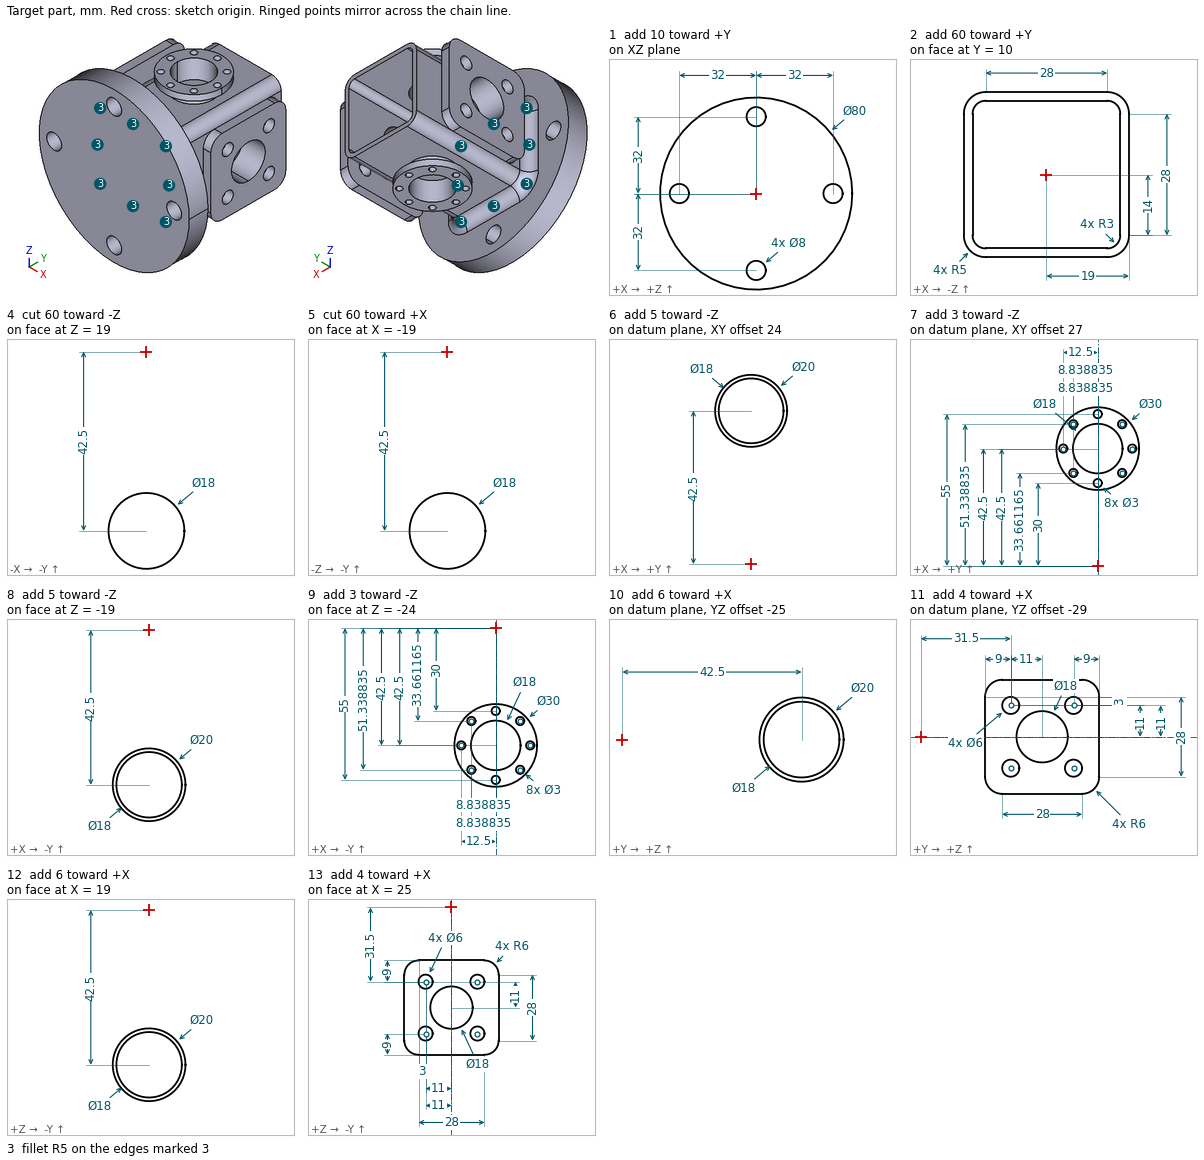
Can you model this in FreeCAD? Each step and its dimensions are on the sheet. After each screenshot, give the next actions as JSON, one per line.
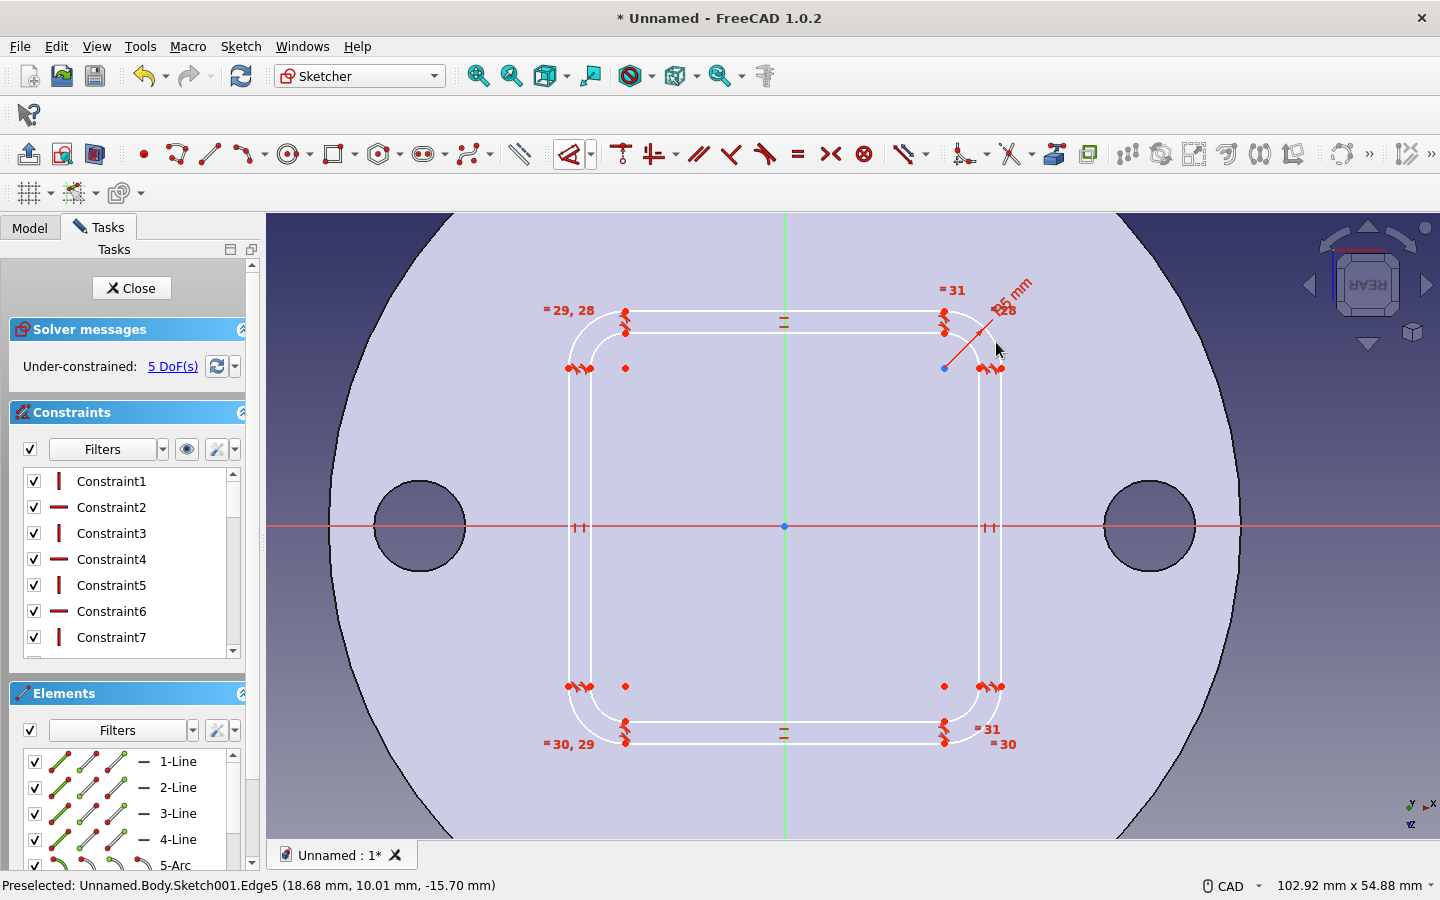
{"action": "left_click", "coordinate": [960, 718]}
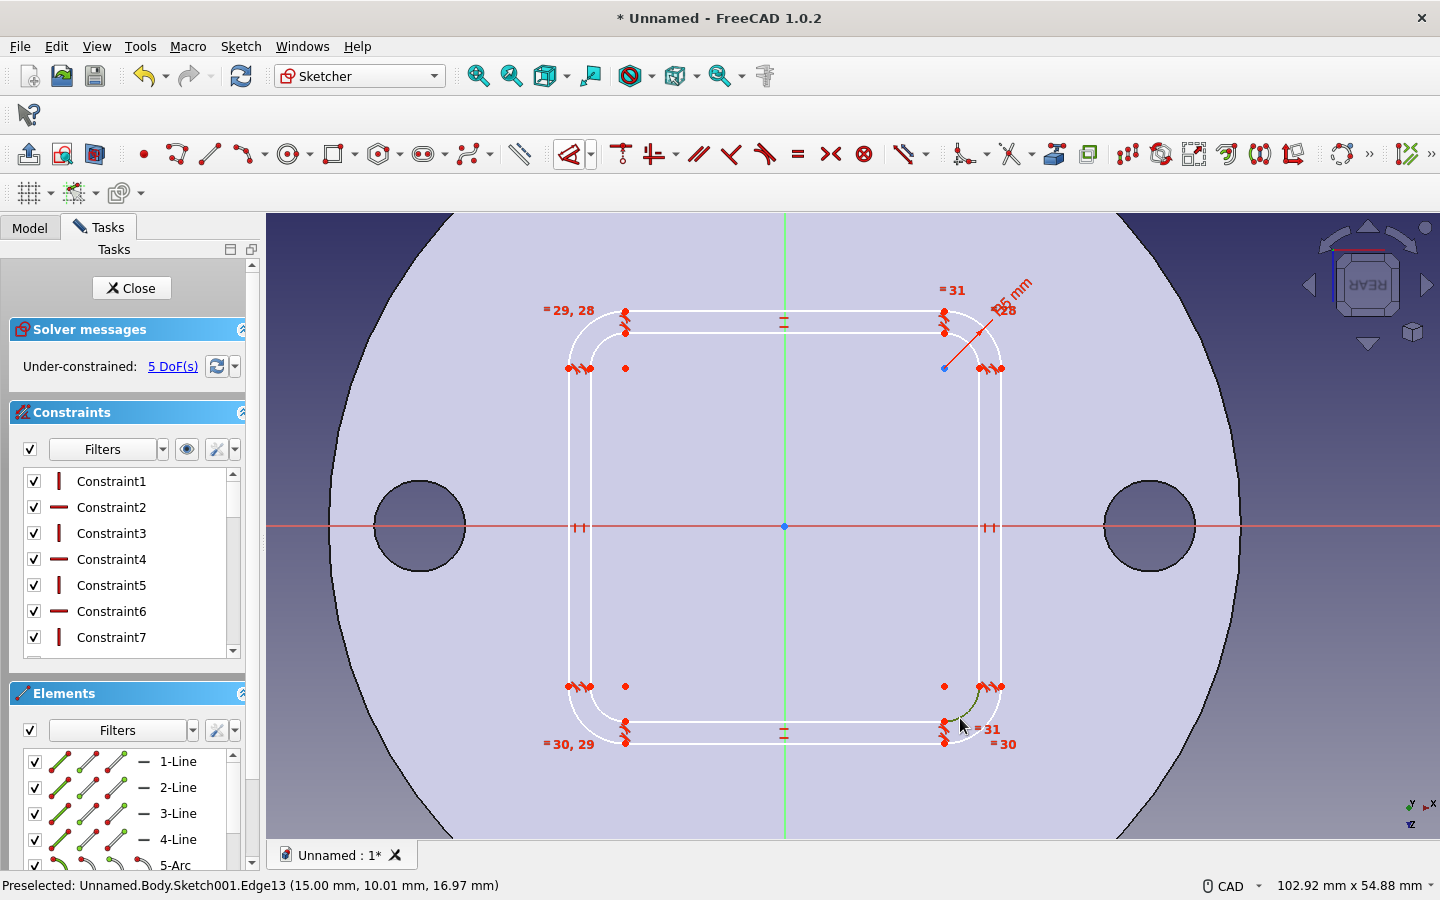
{"action": "key", "text": "k r"}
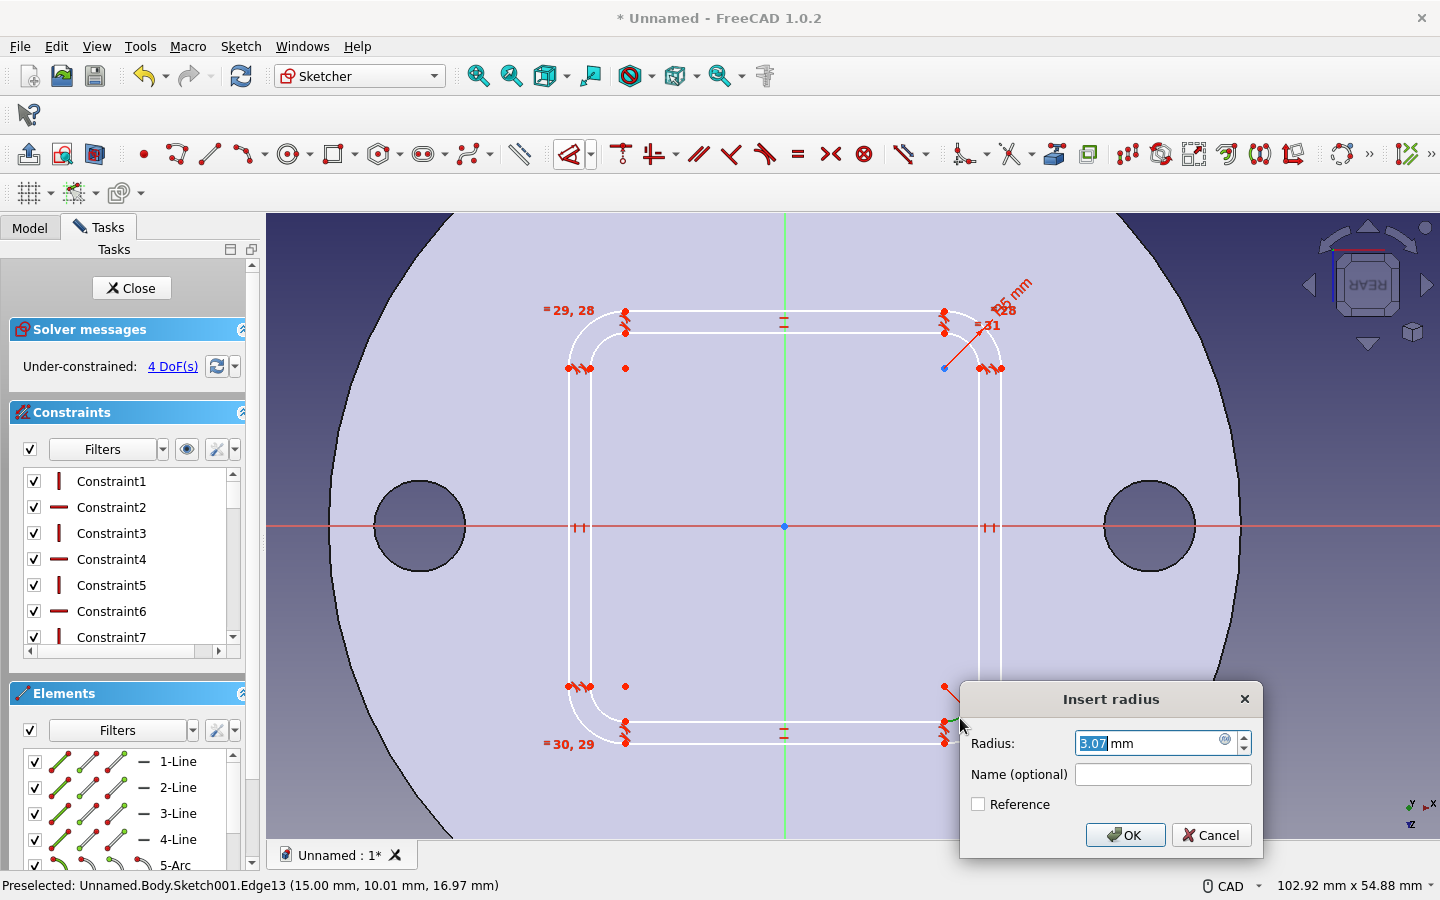
{"action": "type", "text": "3"}
{"action": "key", "text": "Return"}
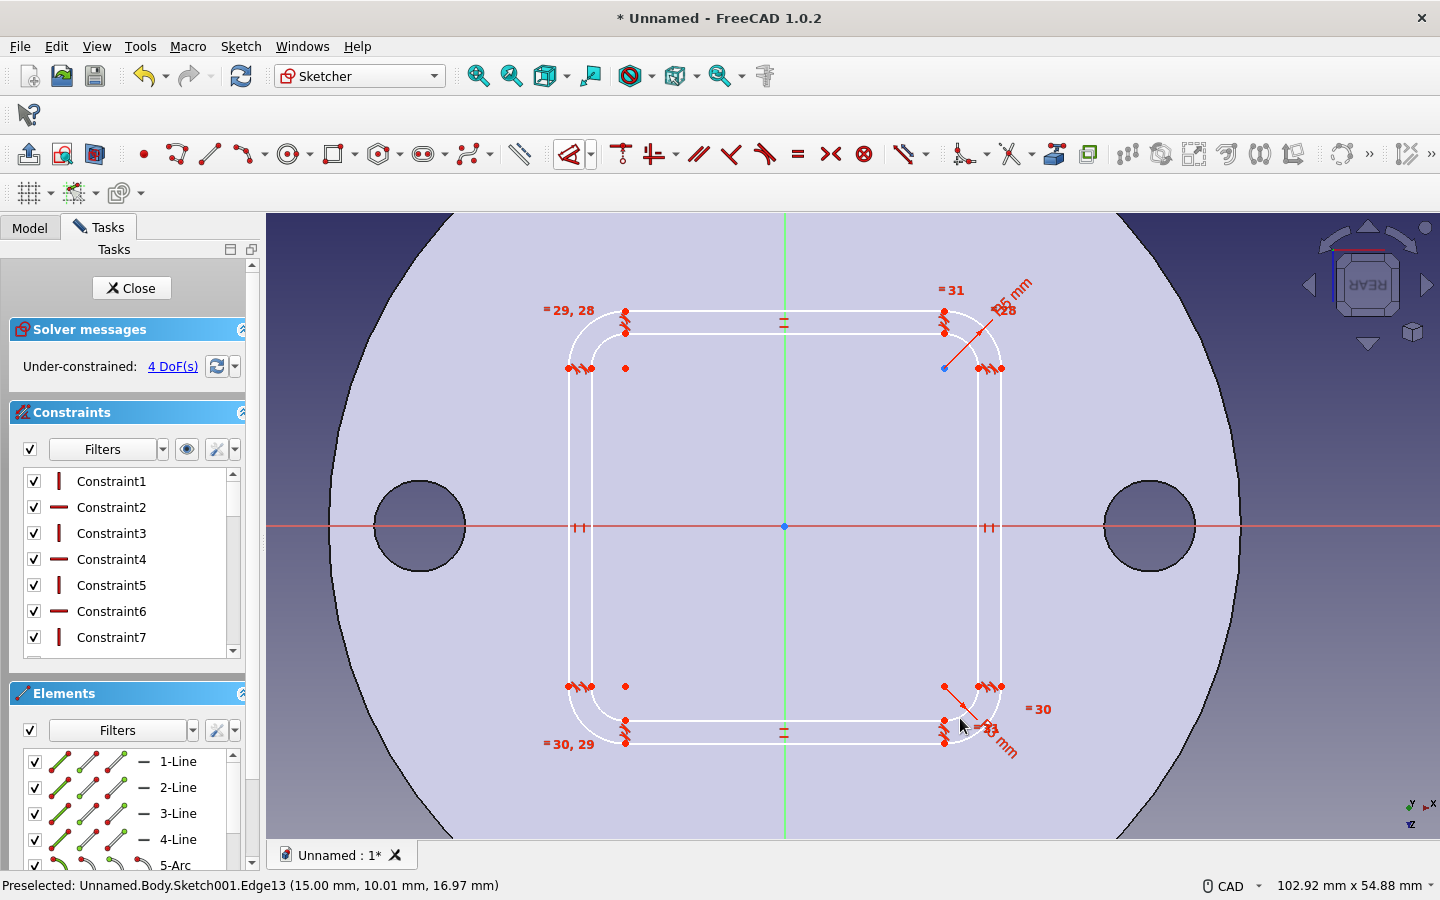
{"action": "left_click", "coordinate": [1001, 591]}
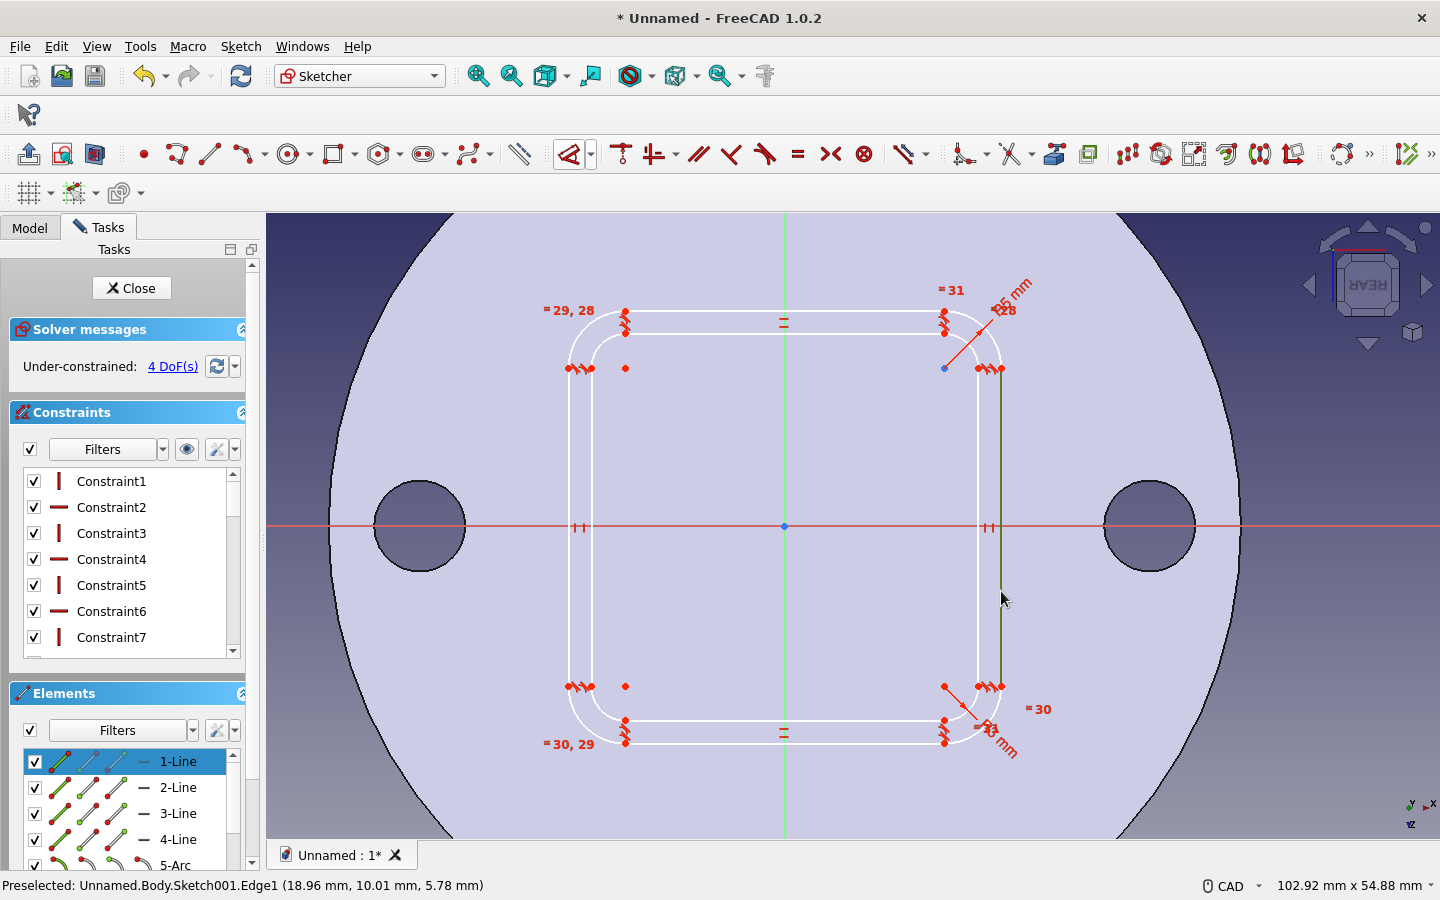
{"action": "key", "text": "i"}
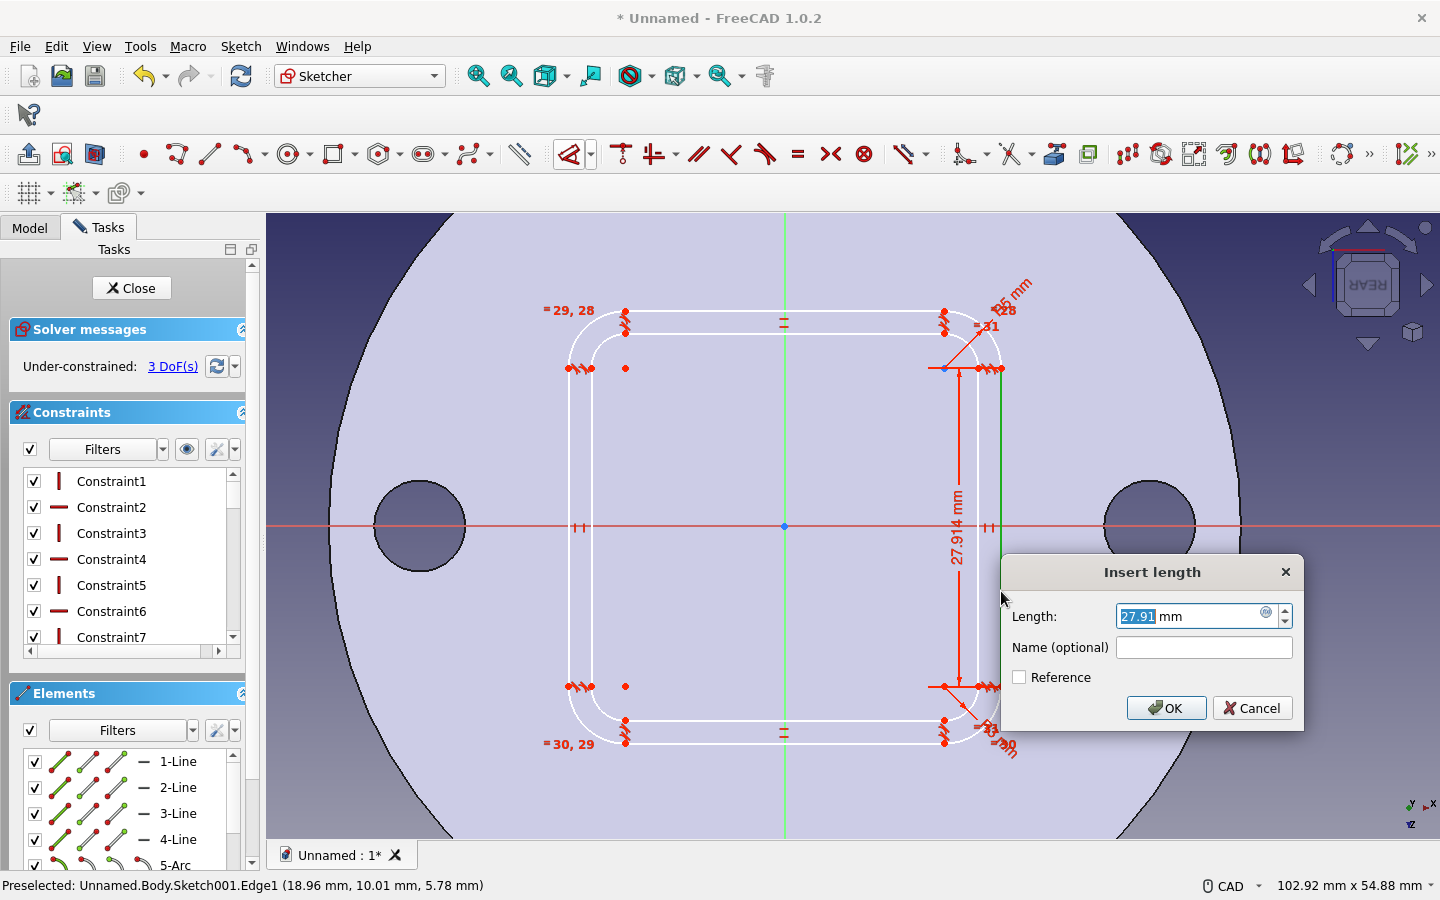
{"action": "type", "text": "28"}
{"action": "key", "text": "Return"}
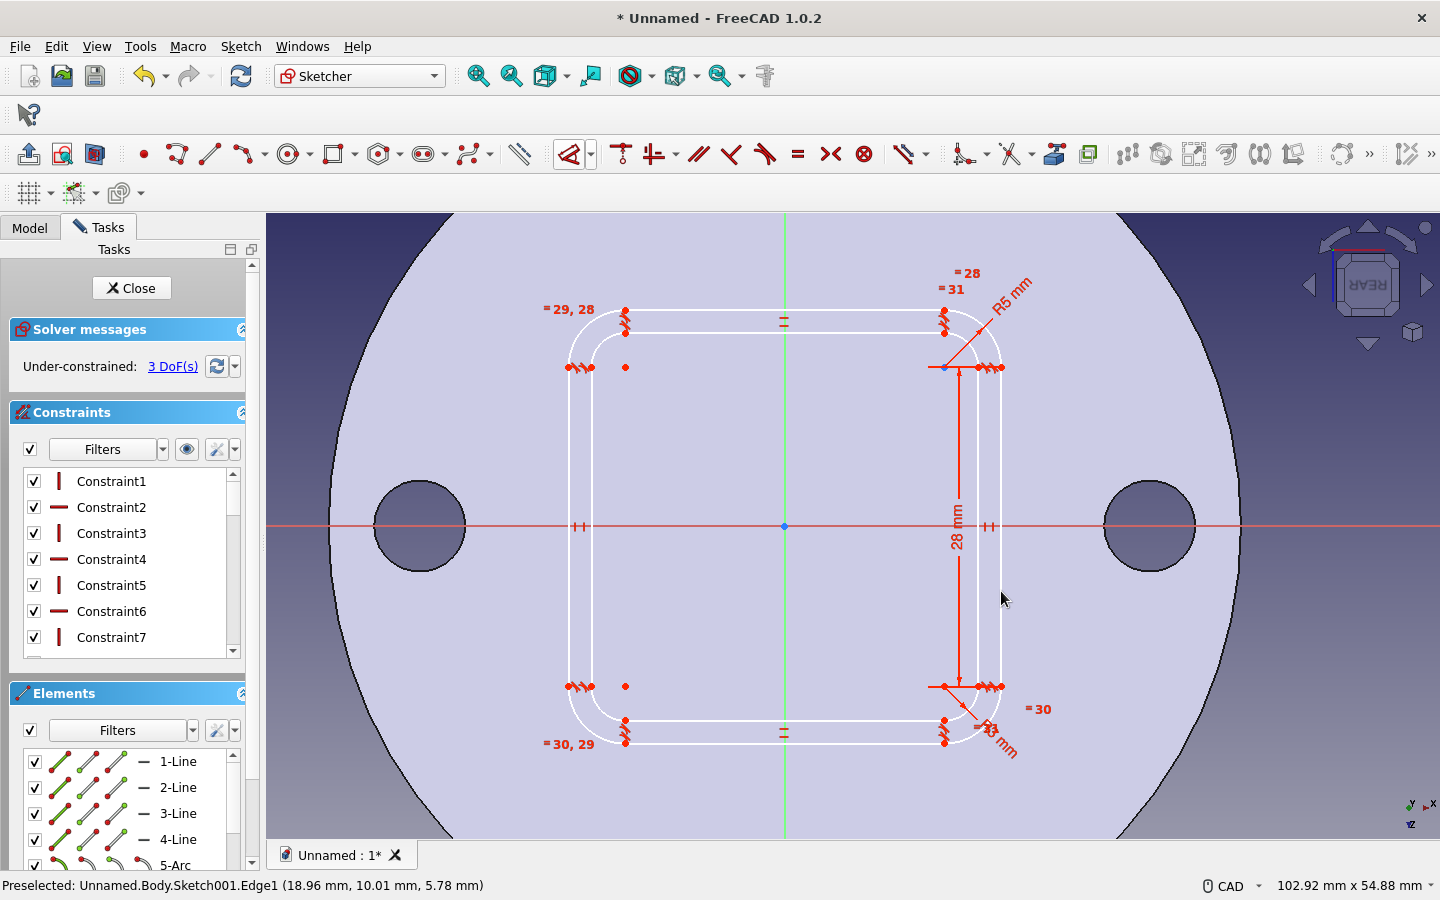
{"action": "left_click", "coordinate": [849, 310]}